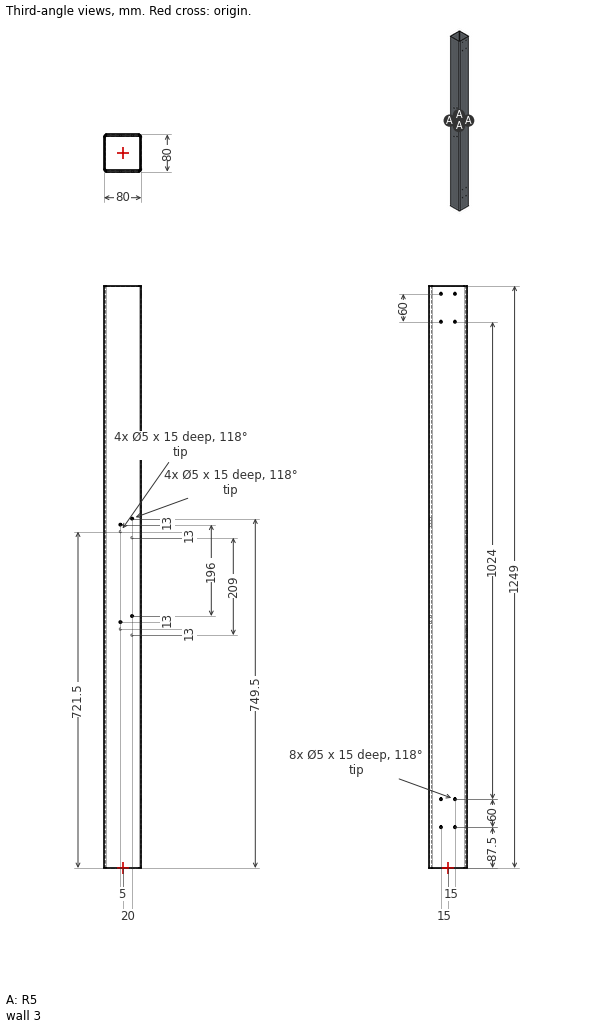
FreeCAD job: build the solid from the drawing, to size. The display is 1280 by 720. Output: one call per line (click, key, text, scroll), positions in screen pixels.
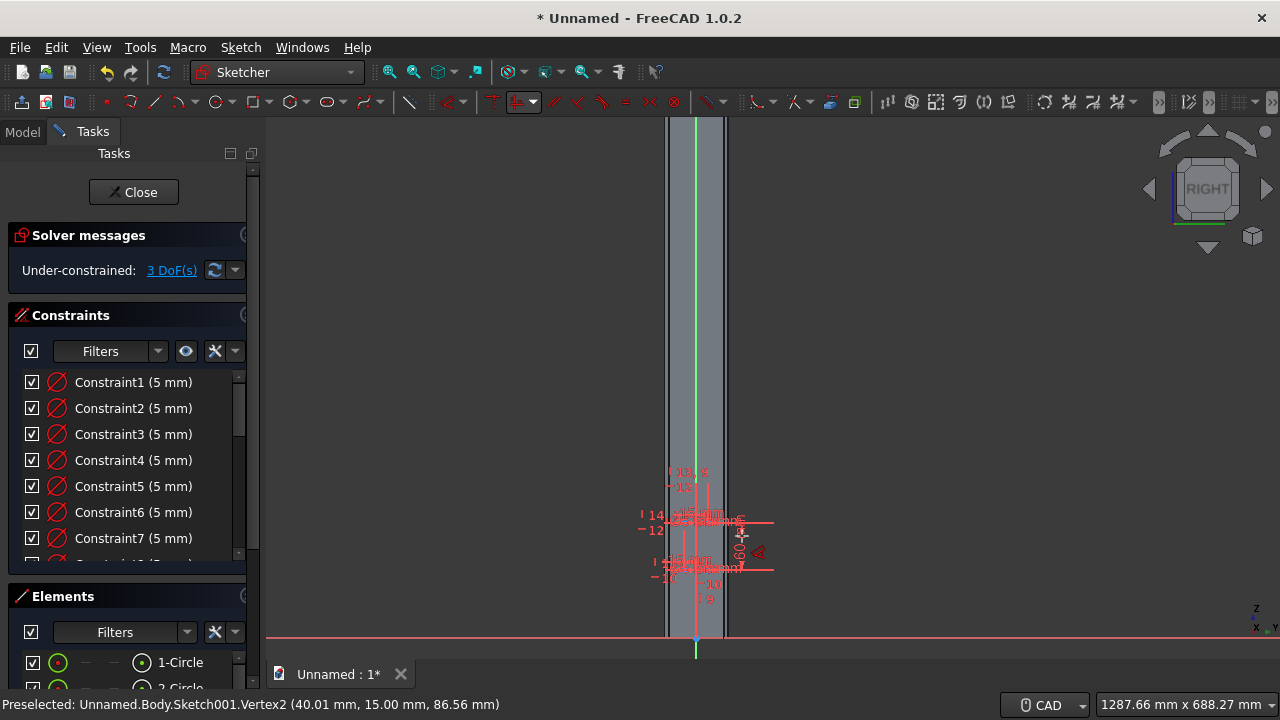
scroll(709, 525, down, 5)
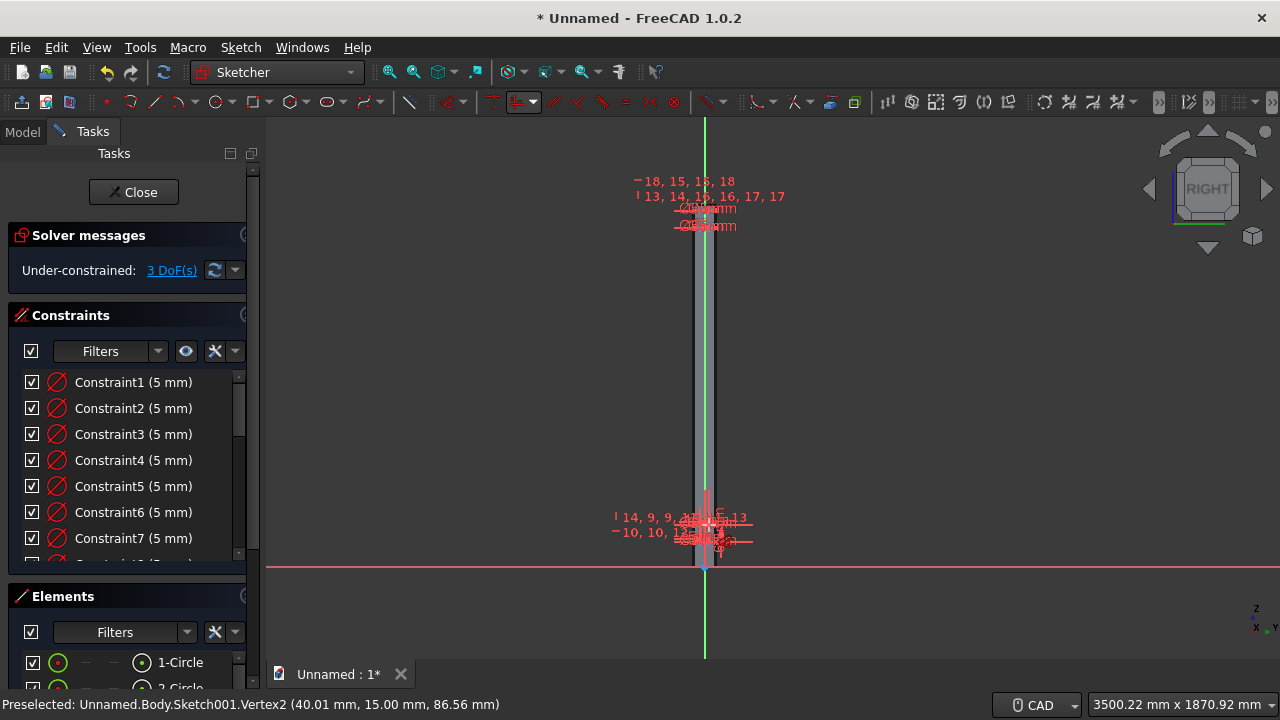
scroll(700, 228, up, 5)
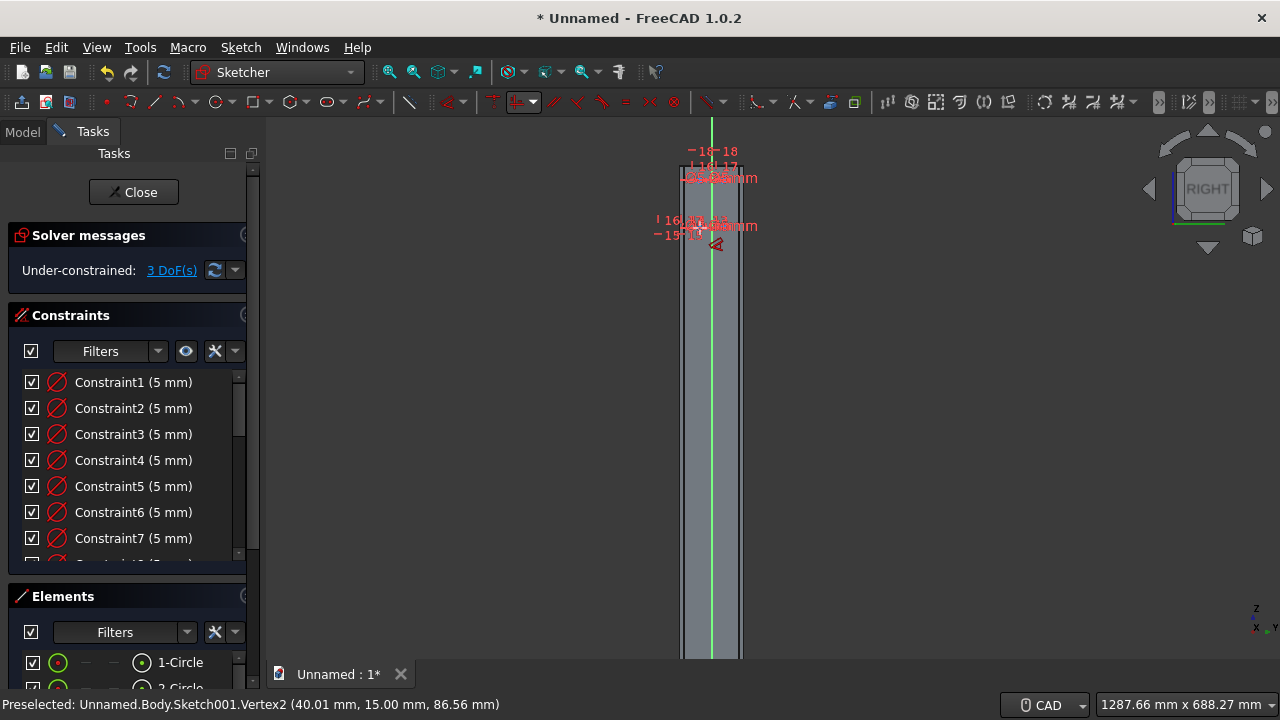
click(700, 228)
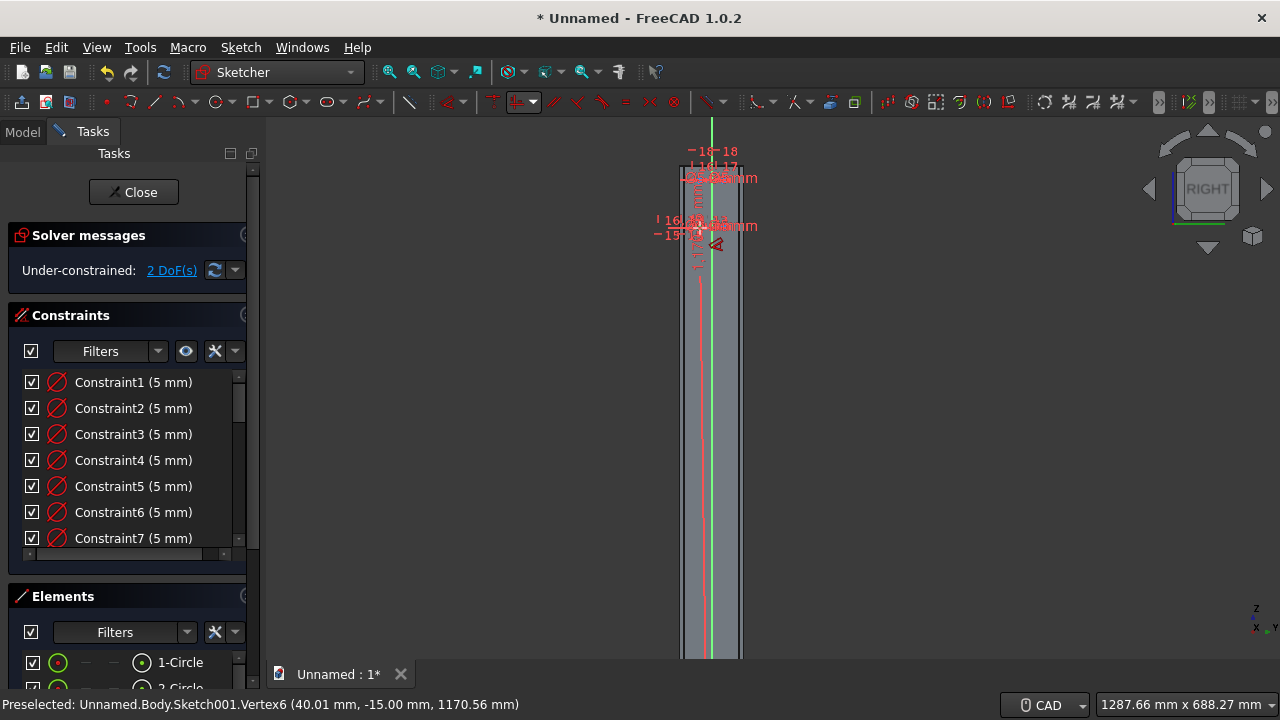
click(700, 180)
click(666, 204)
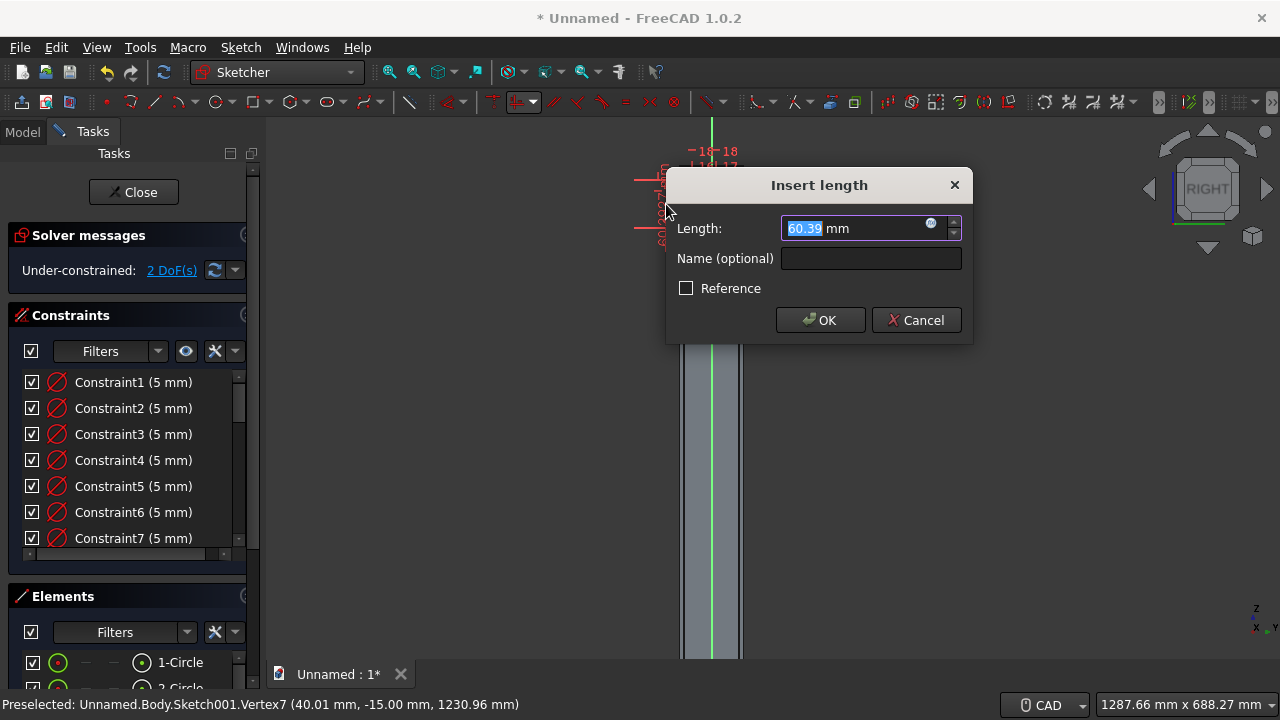
text(60)
key(Return)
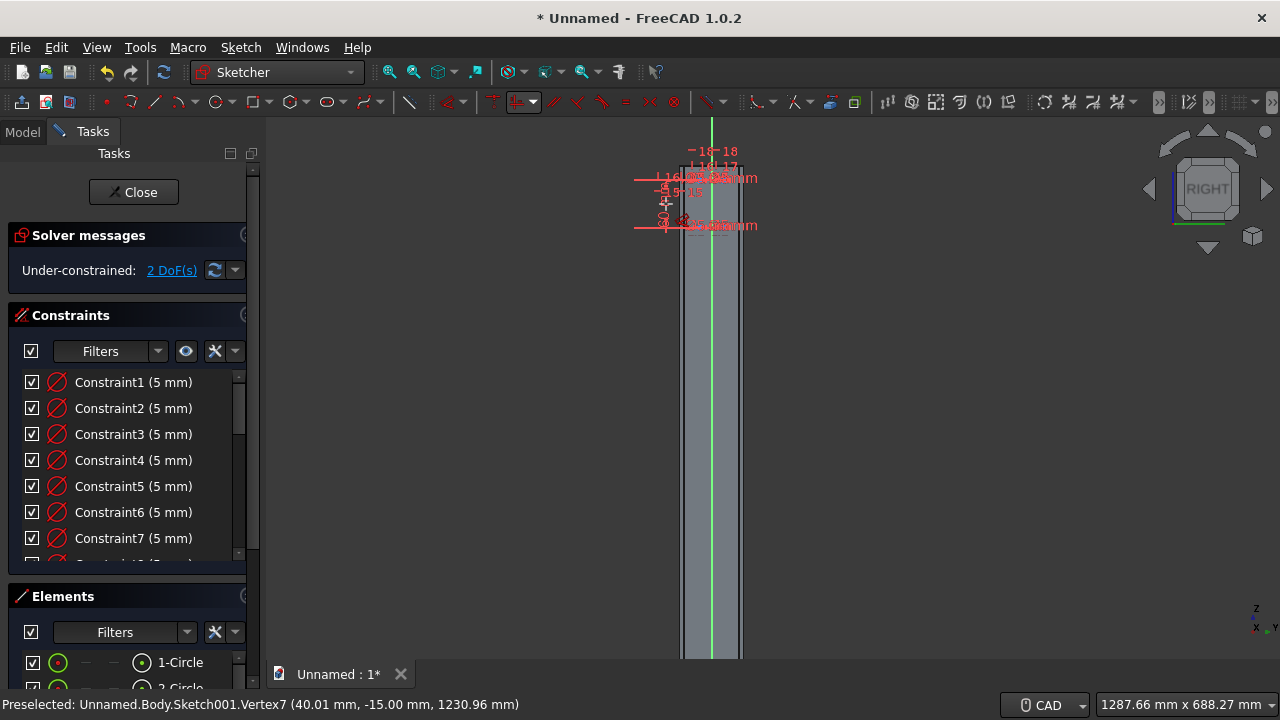
scroll(700, 228, down, 5)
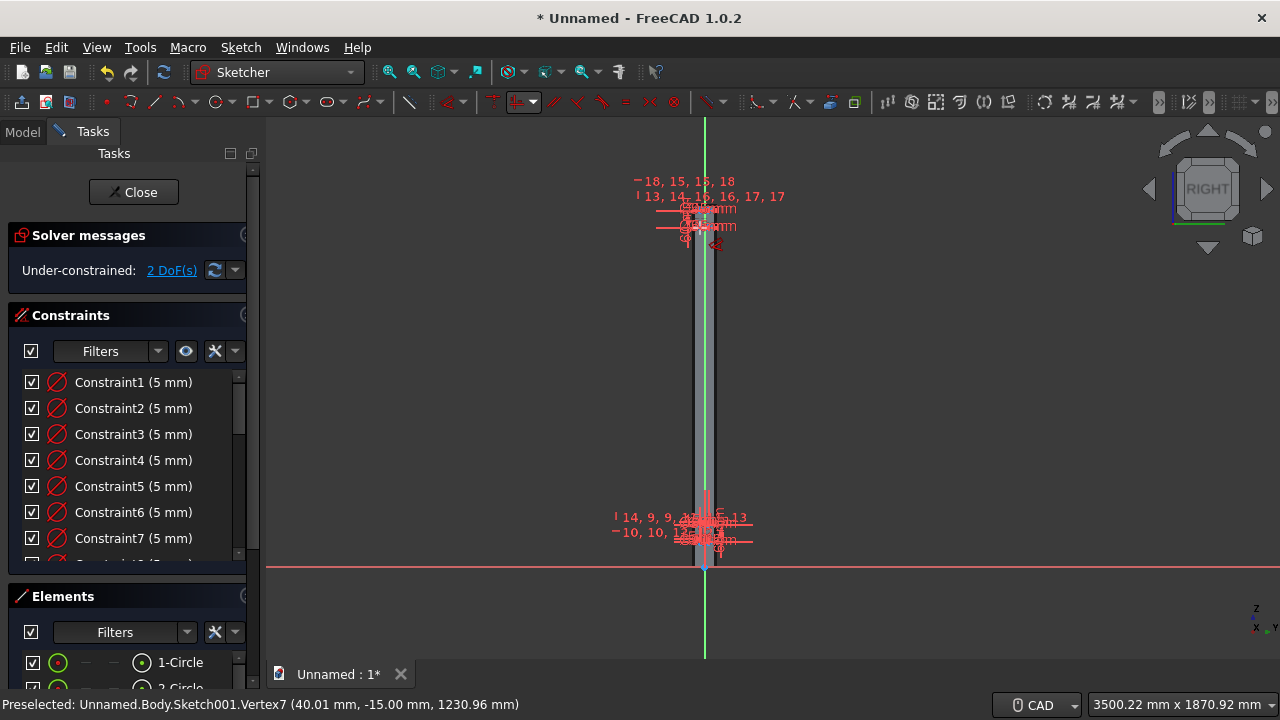
scroll(709, 542, up, 3)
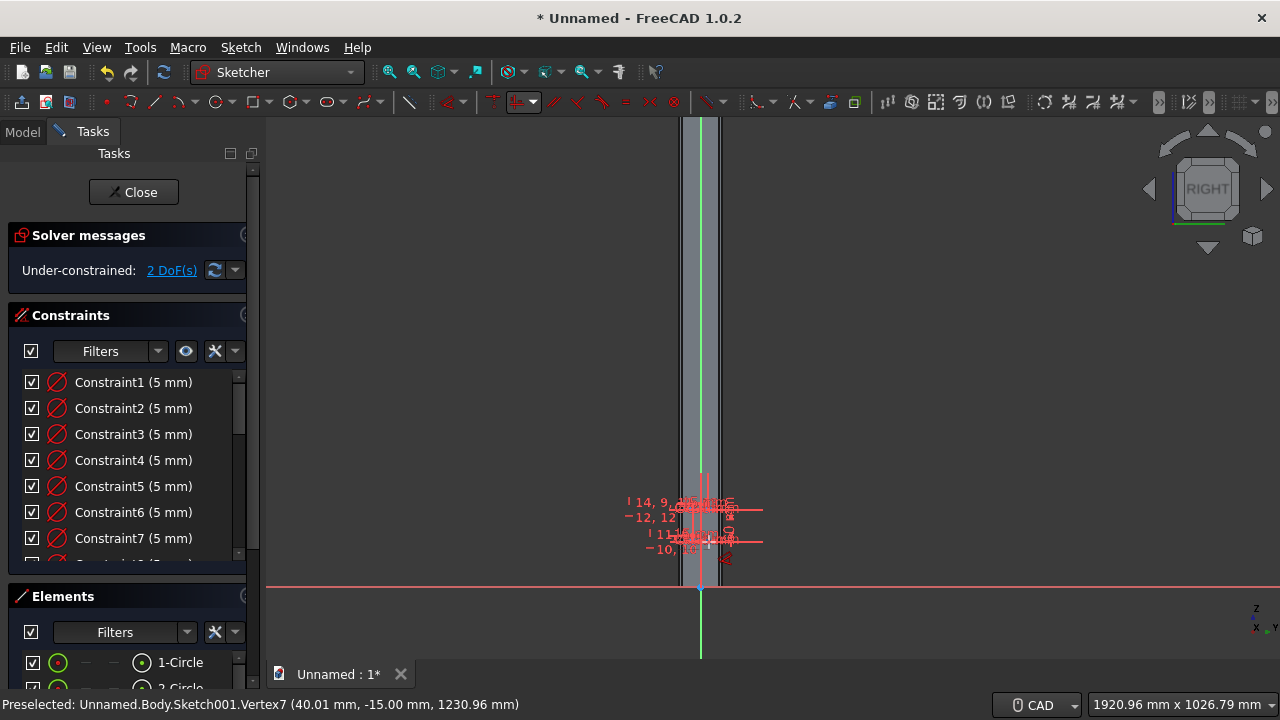
click(708, 542)
click(742, 564)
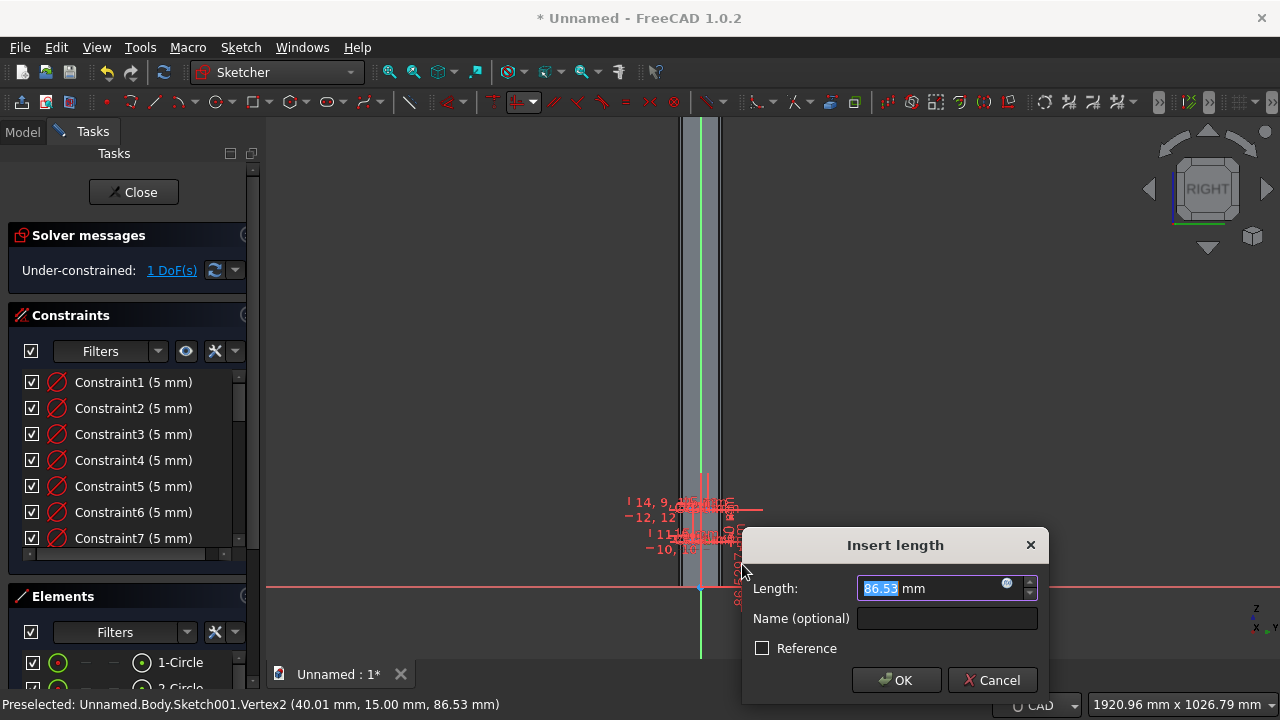
text(87.5)
key(Return)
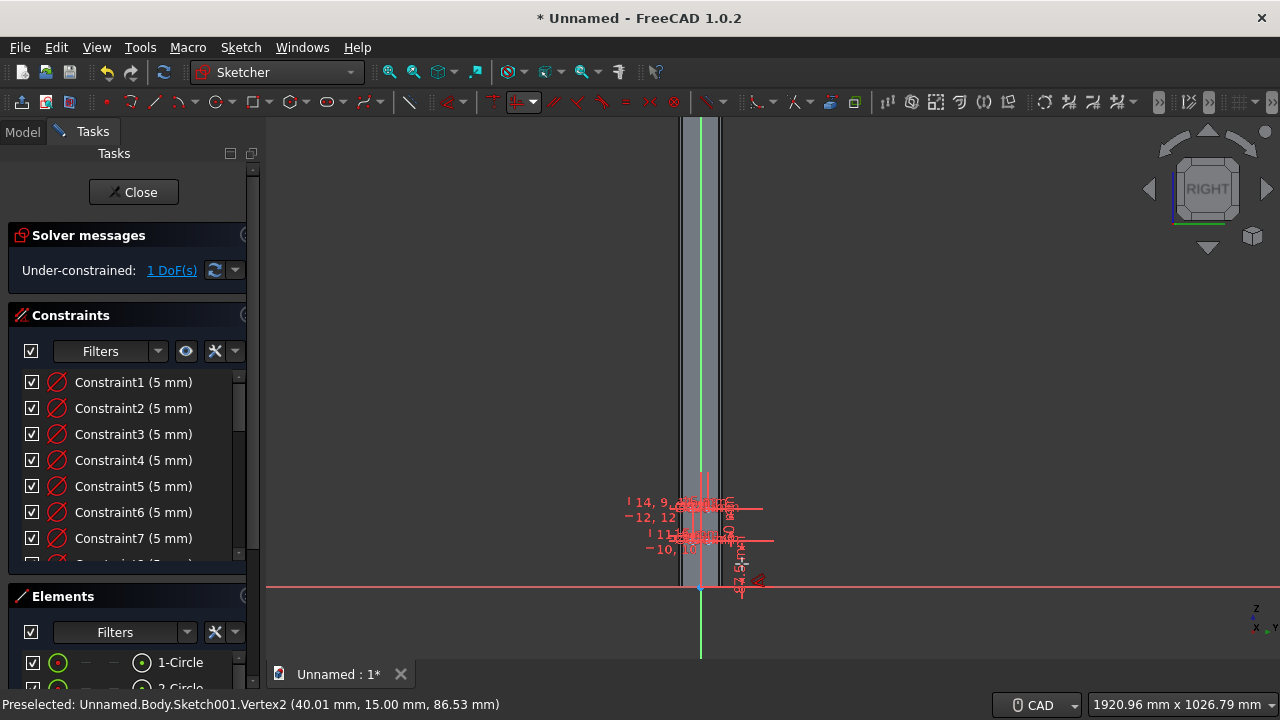
click(708, 509)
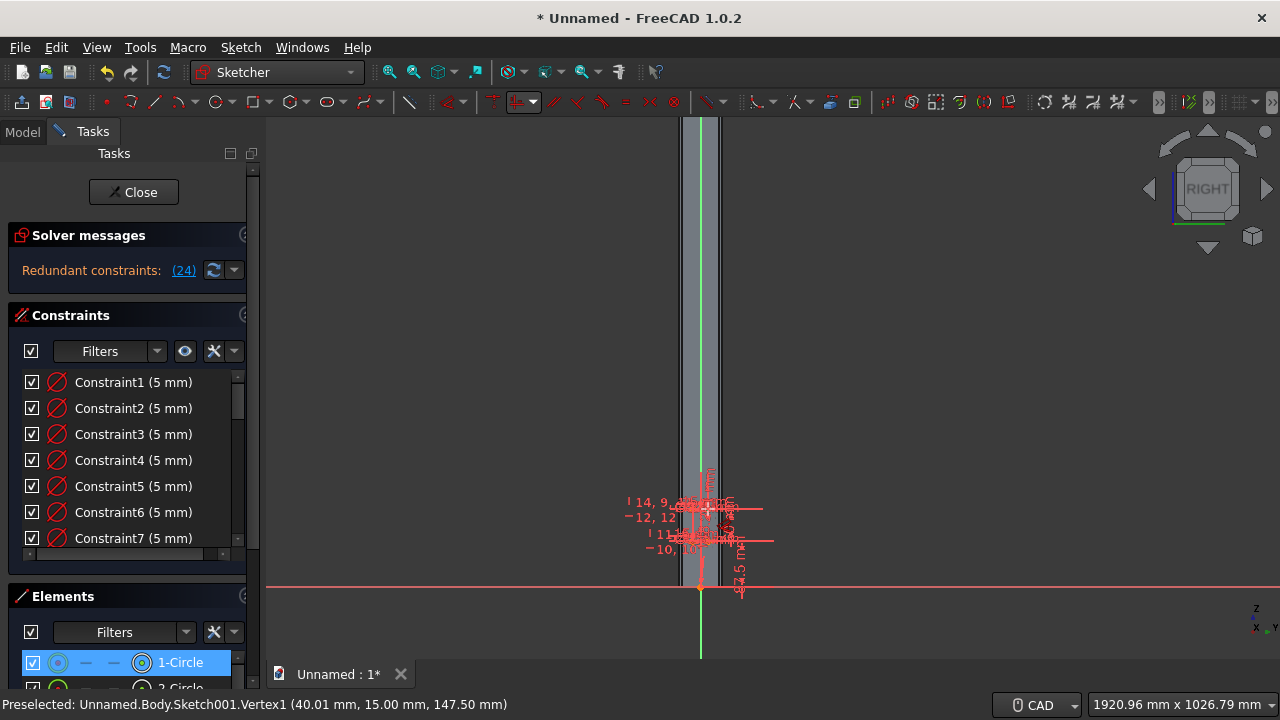
scroll(709, 542, down, 3)